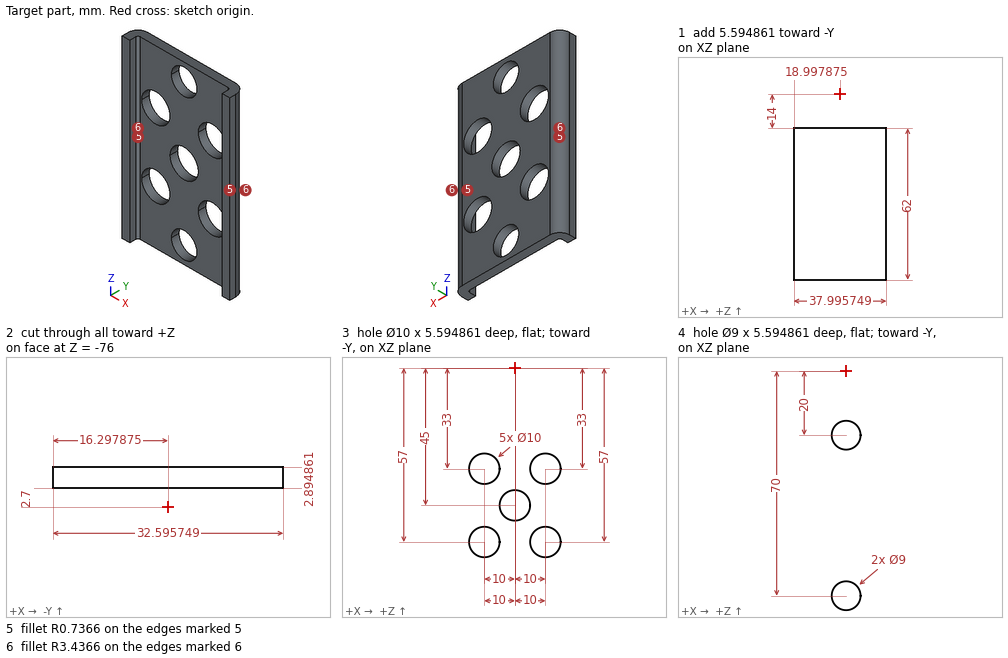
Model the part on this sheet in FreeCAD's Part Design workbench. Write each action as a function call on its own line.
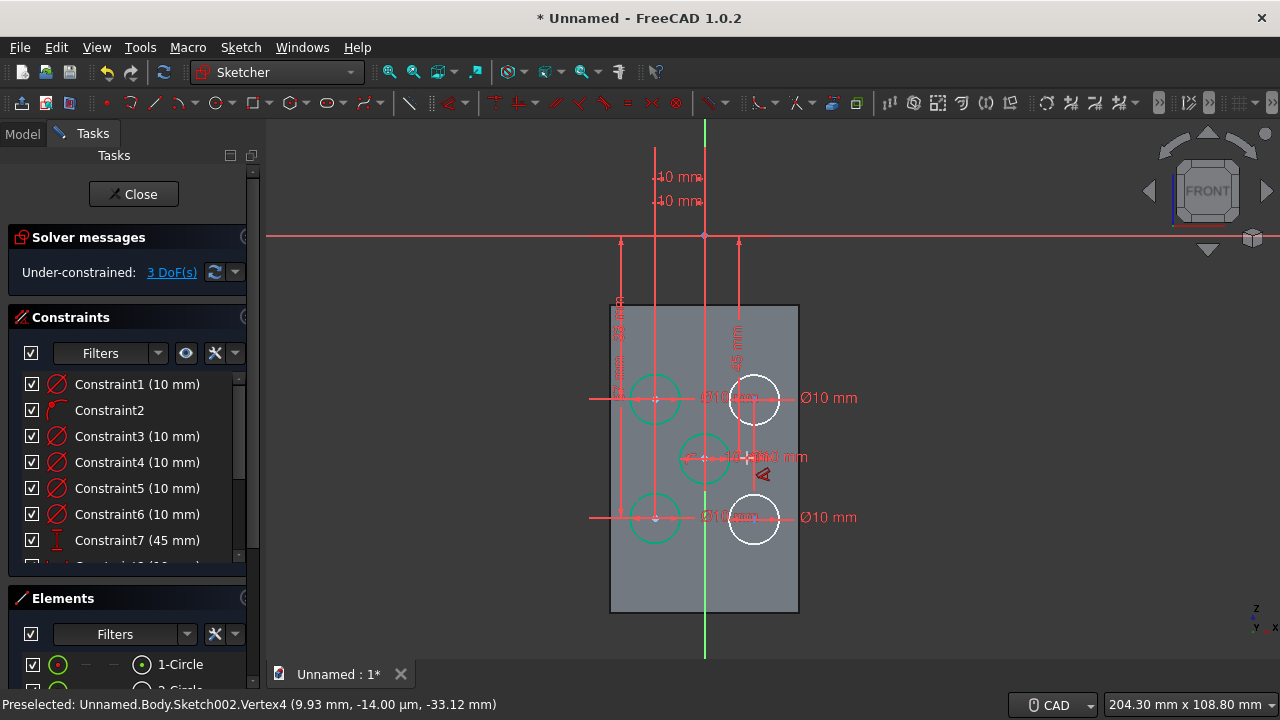
click(754, 400)
click(788, 318)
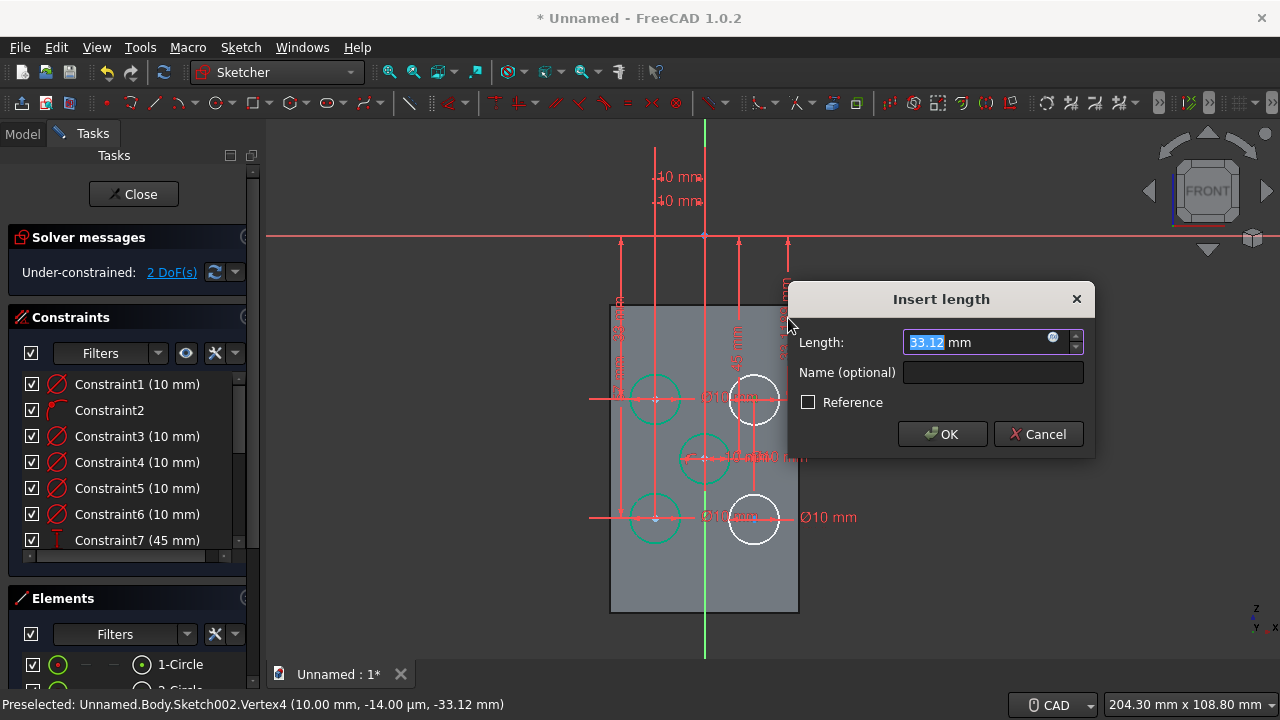
text(33)
key(Return)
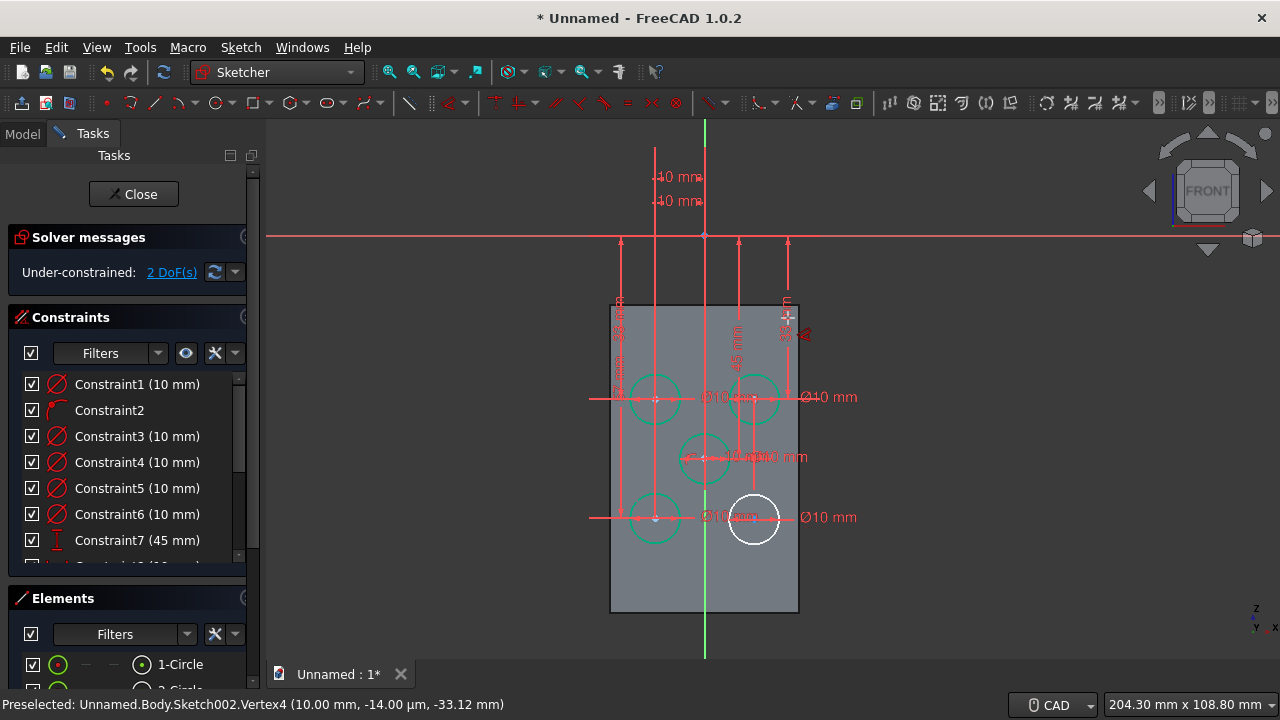
click(754, 520)
click(729, 554)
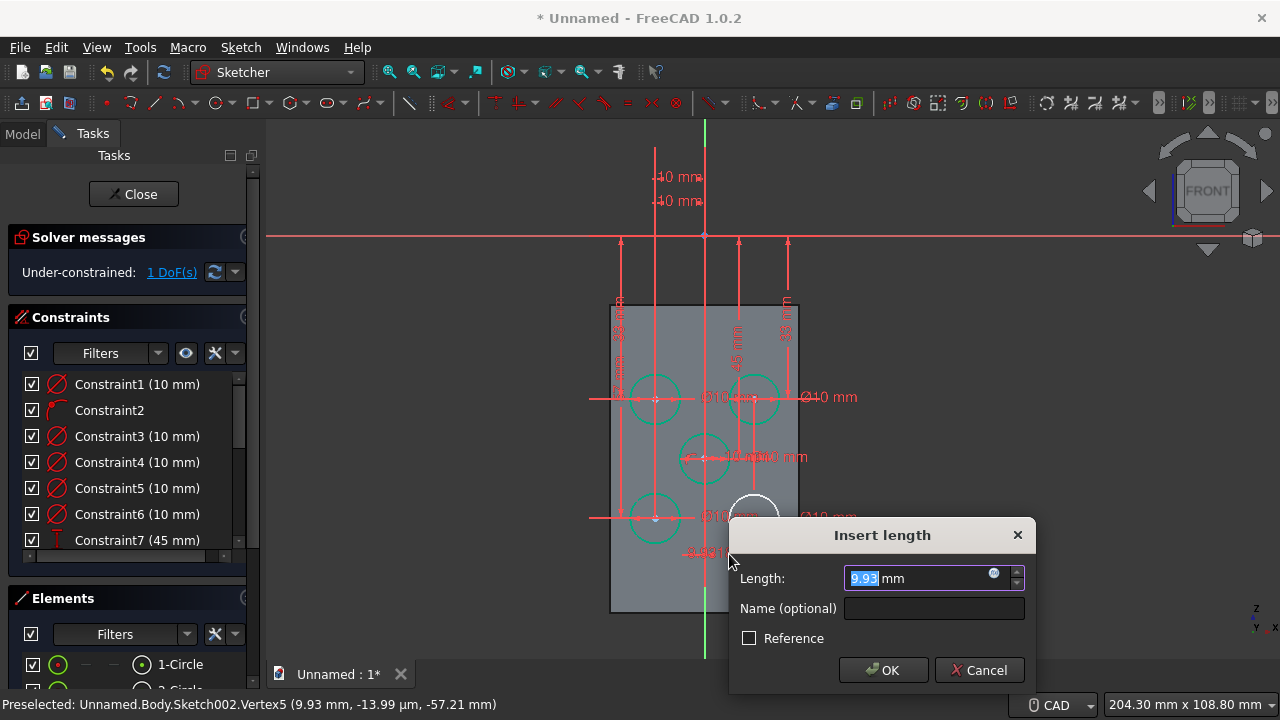
text(10)
key(Return)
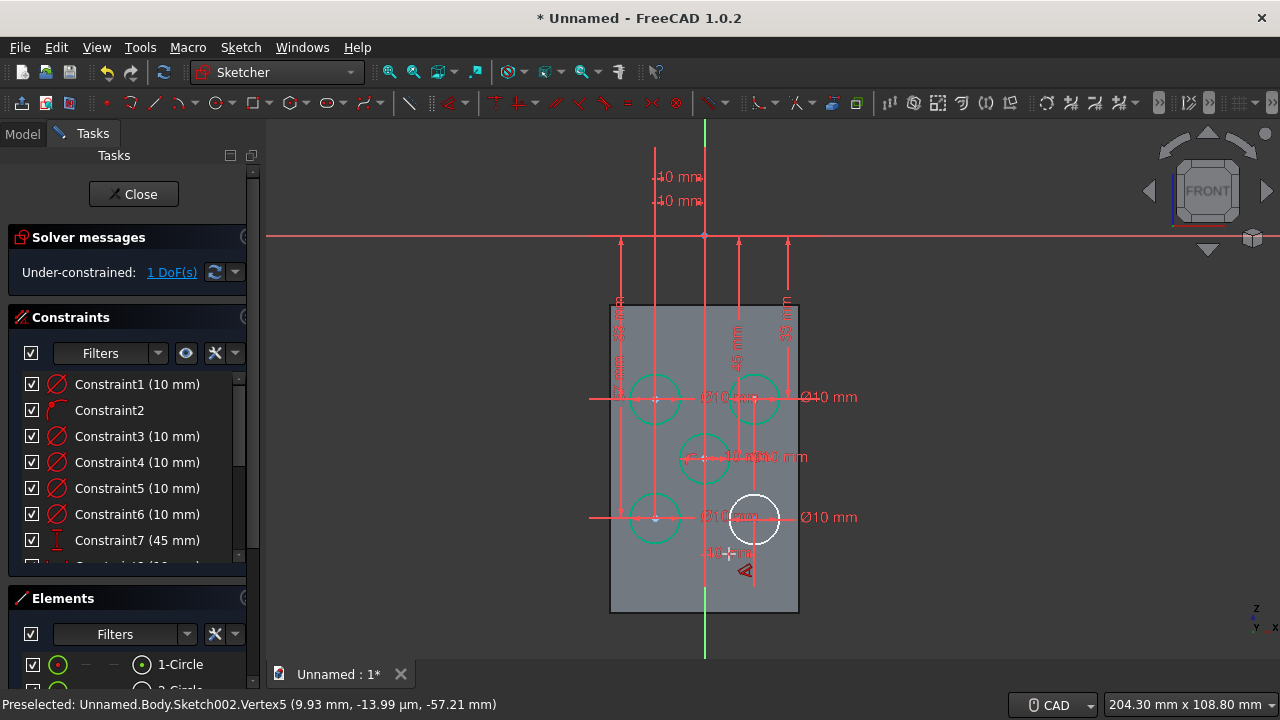
click(754, 520)
click(788, 378)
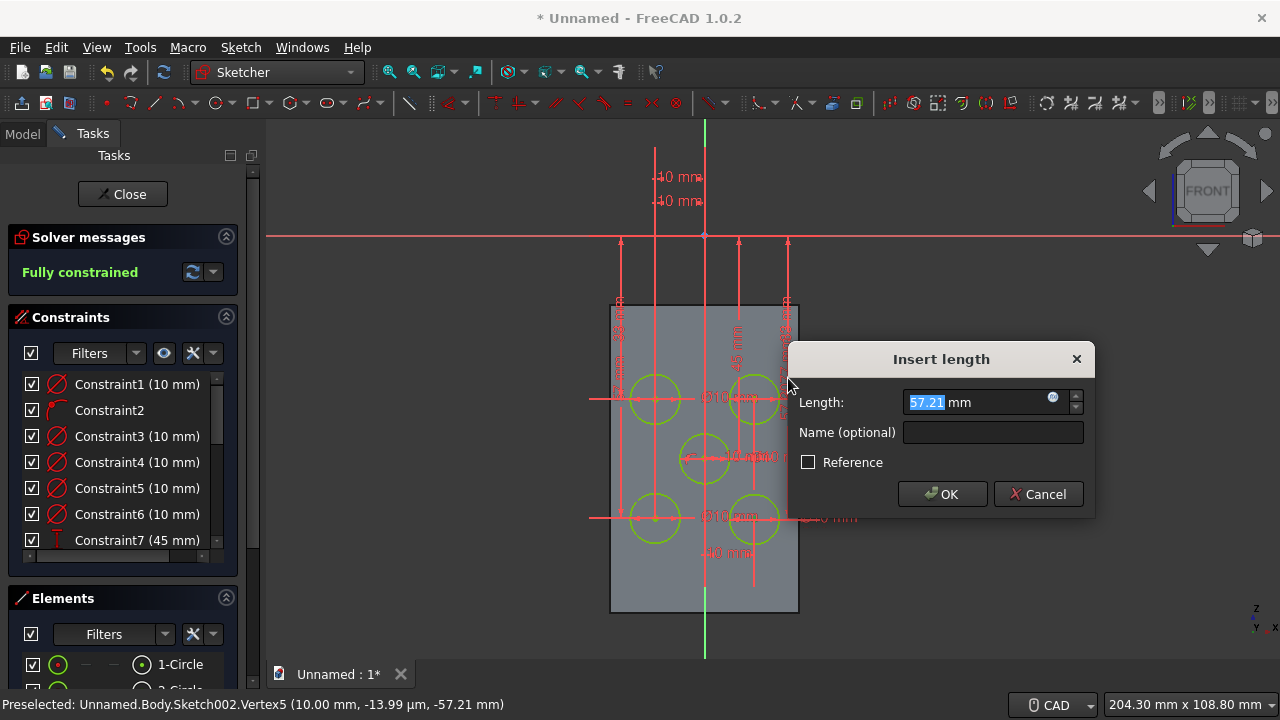
text(57)
key(Return)
key(Escape)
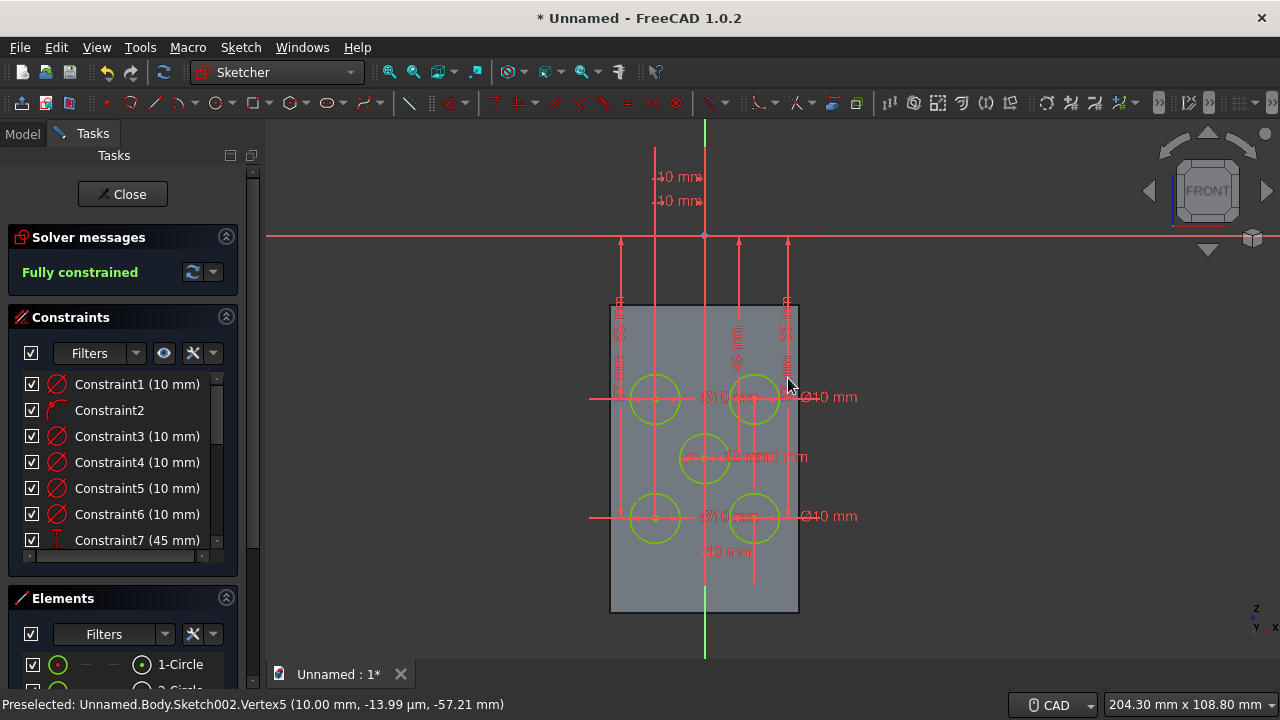
click(123, 194)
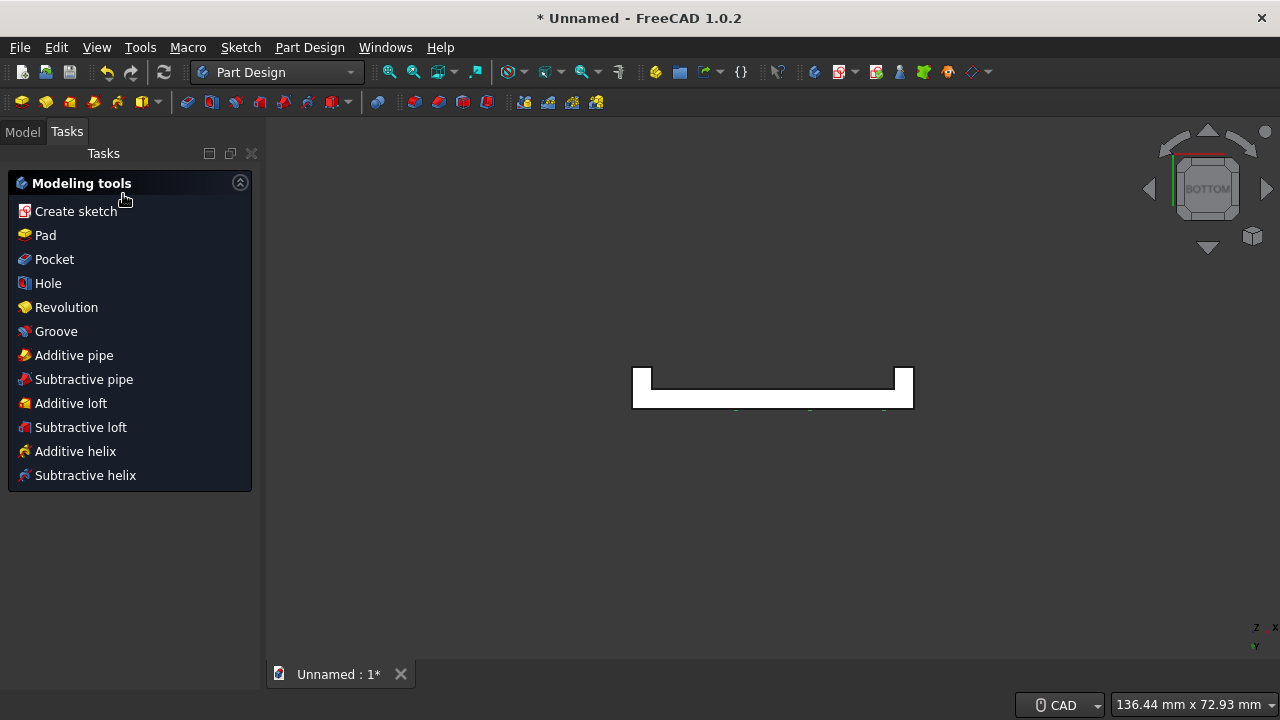
click(212, 102)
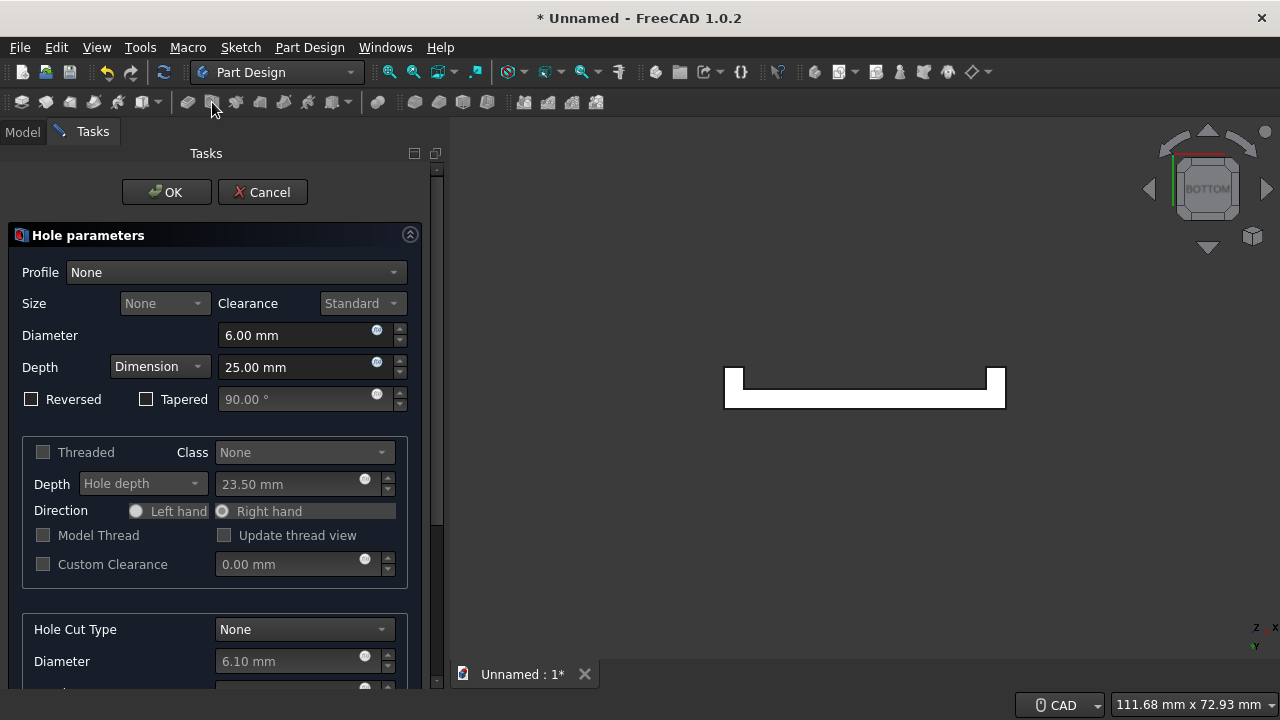
triple_click(305, 335)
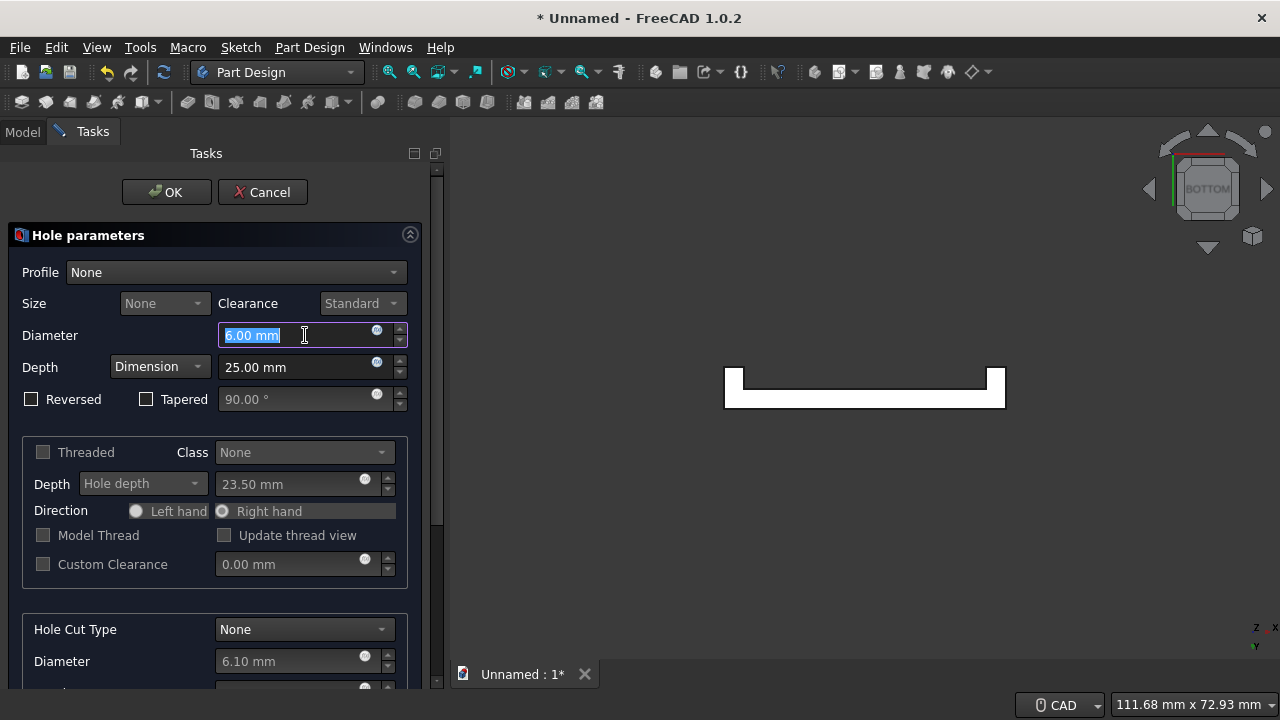
text(10)
key(Tab)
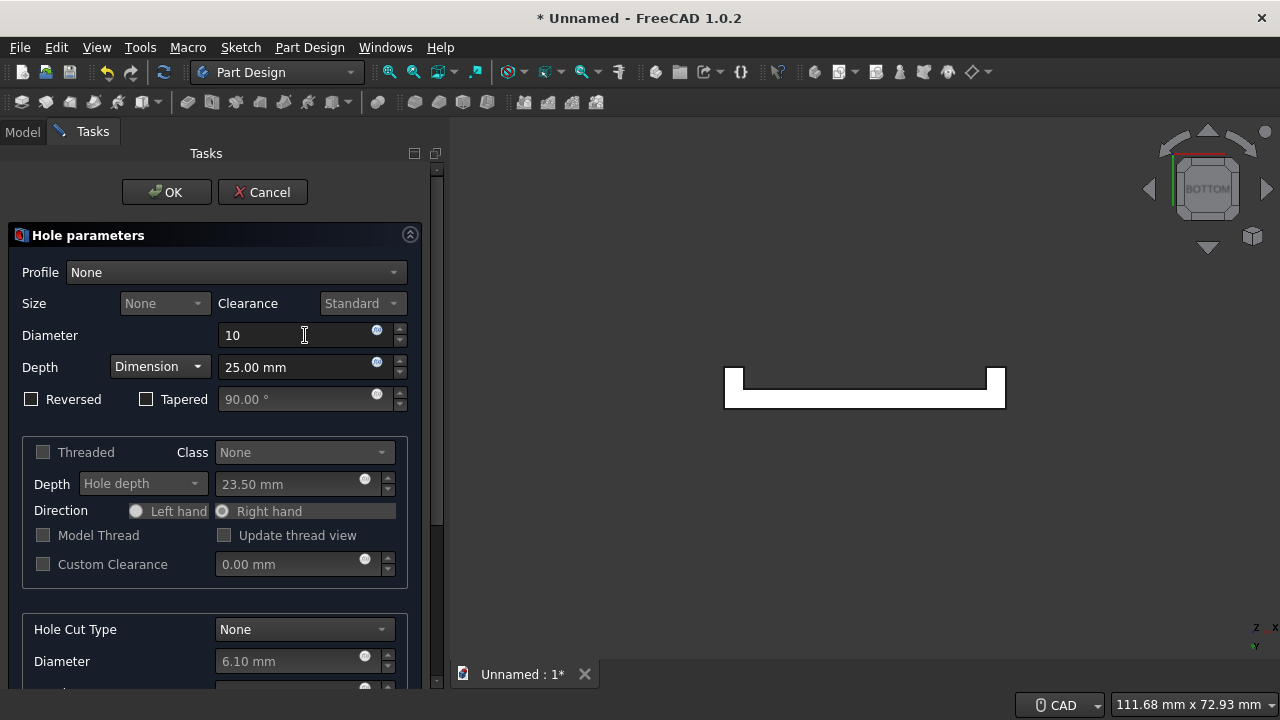
triple_click(305, 367)